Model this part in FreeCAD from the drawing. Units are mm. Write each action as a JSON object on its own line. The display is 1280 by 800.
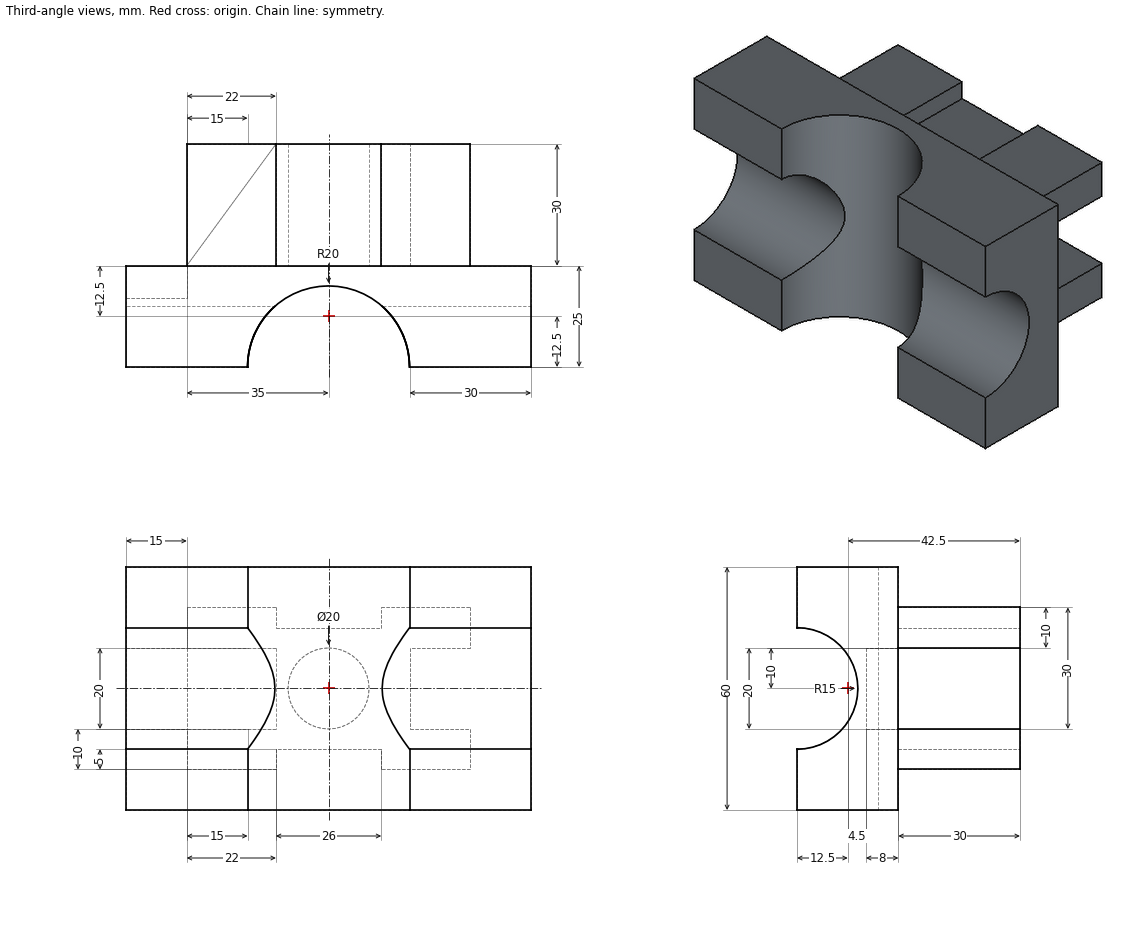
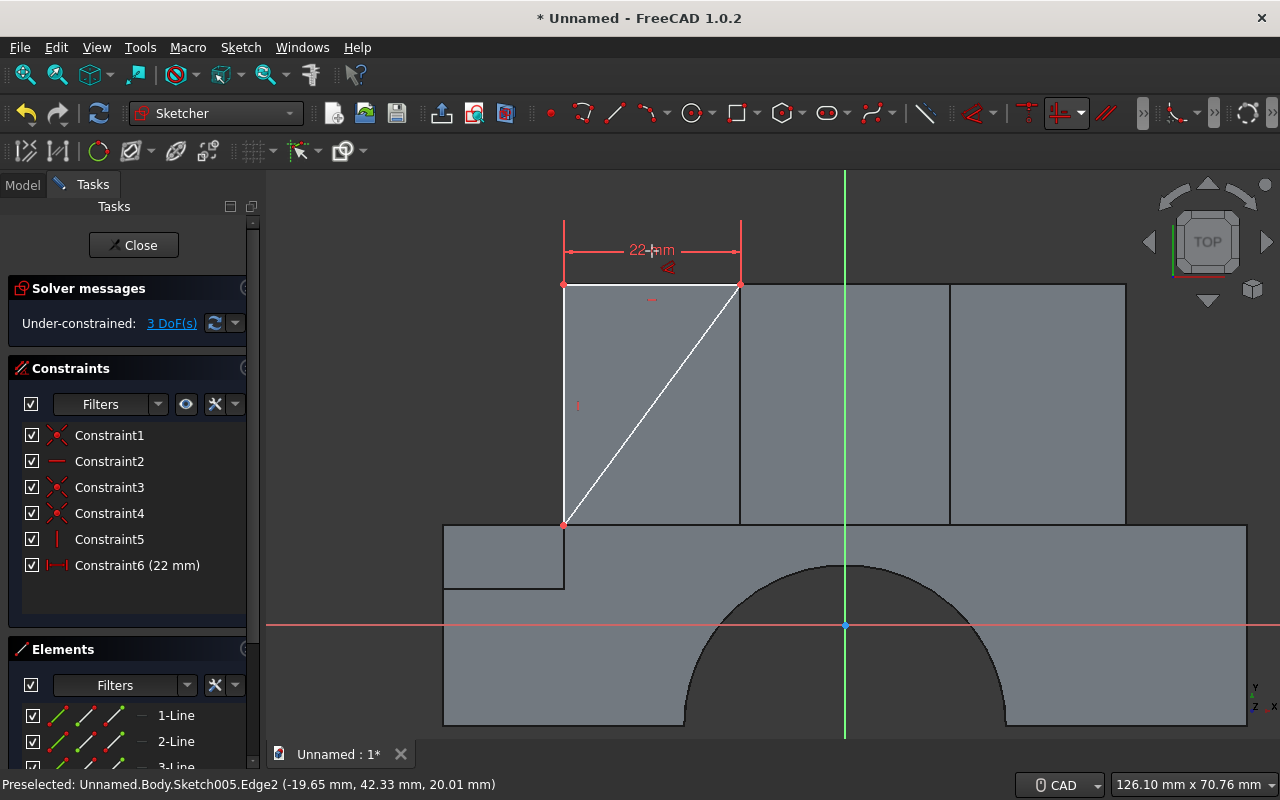
{"action": "left_click", "coordinate": [564, 357]}
{"action": "left_click", "coordinate": [530, 405]}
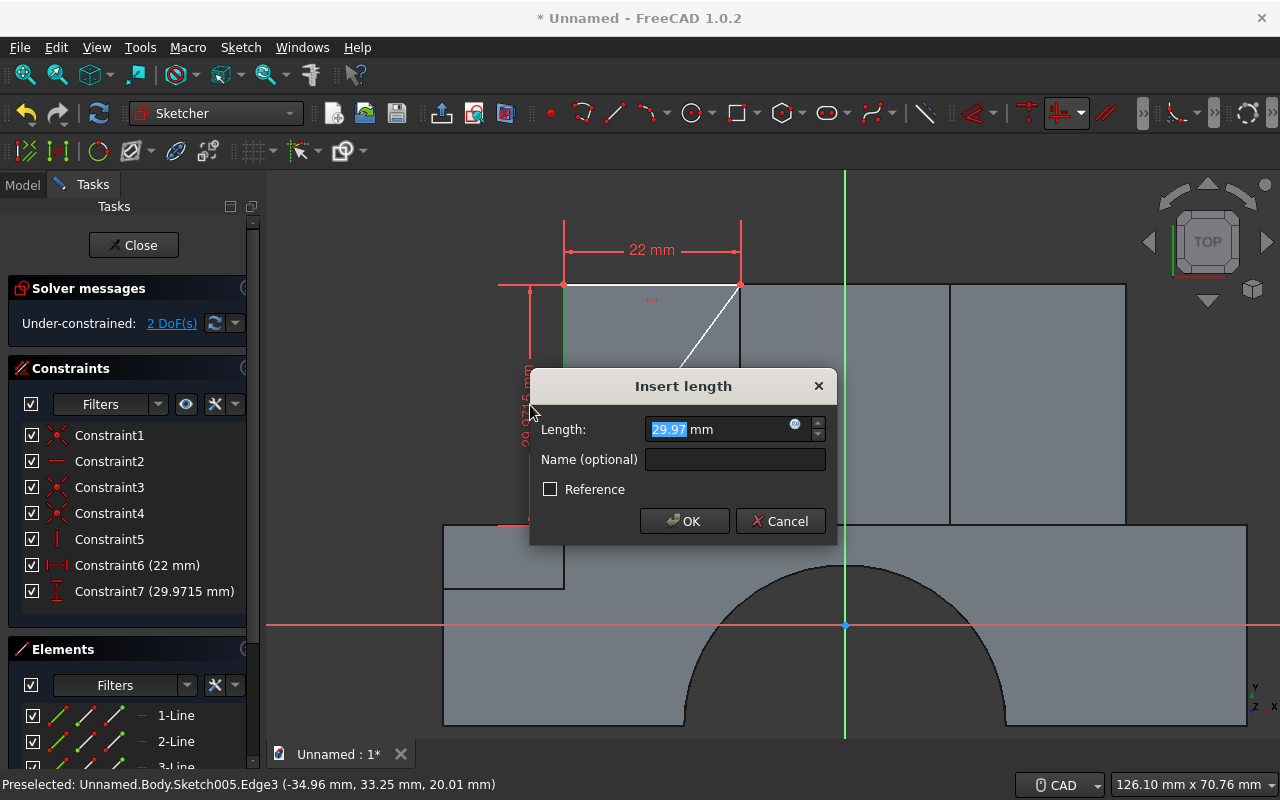
{"action": "type", "text": "30"}
{"action": "key", "text": "Return"}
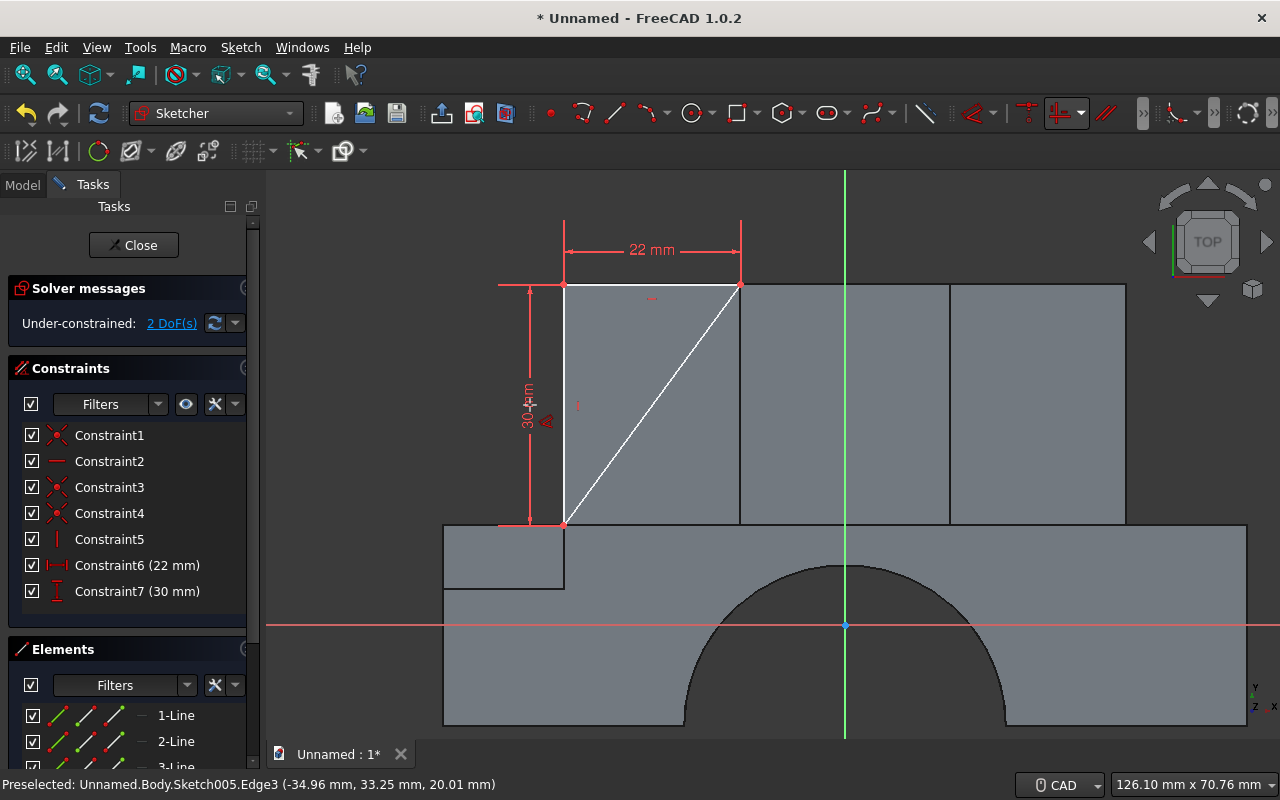
{"action": "left_click", "coordinate": [564, 526]}
{"action": "left_click", "coordinate": [704, 659]}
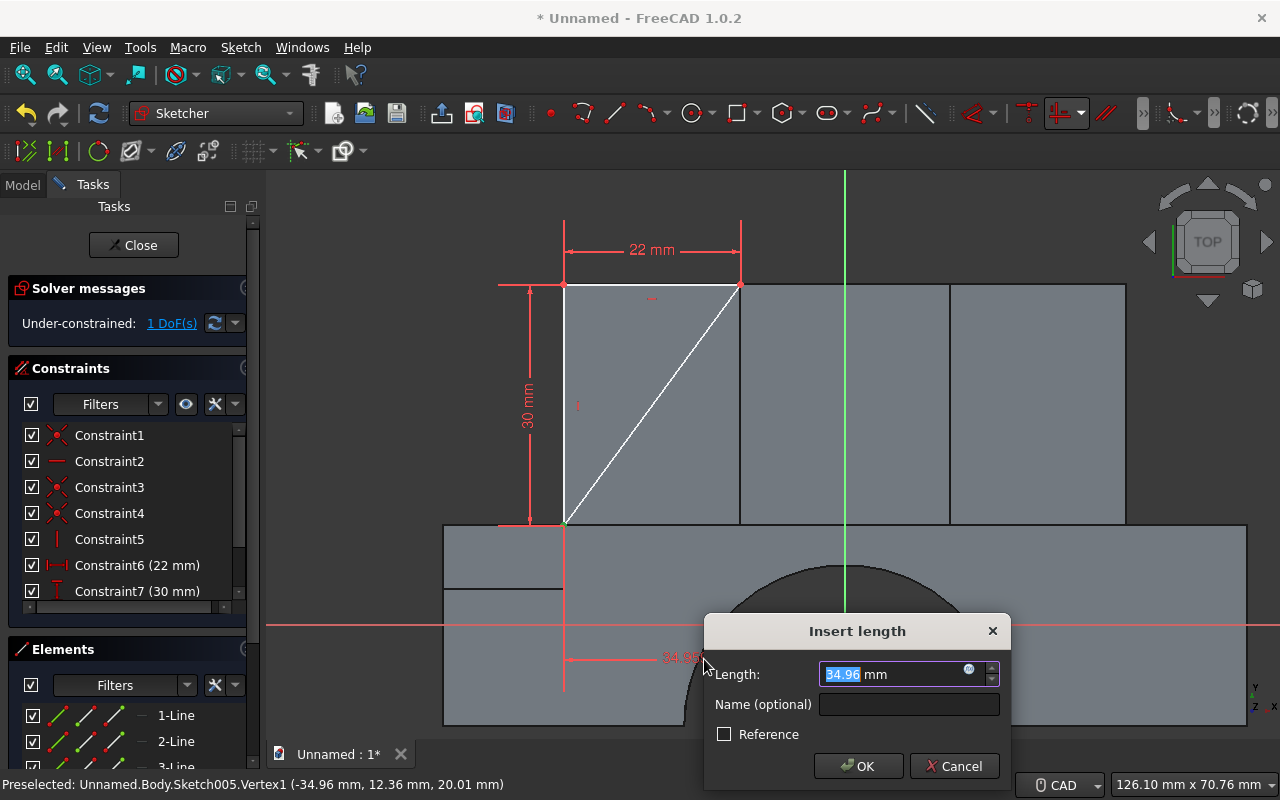
{"action": "type", "text": "35"}
{"action": "key", "text": "Return"}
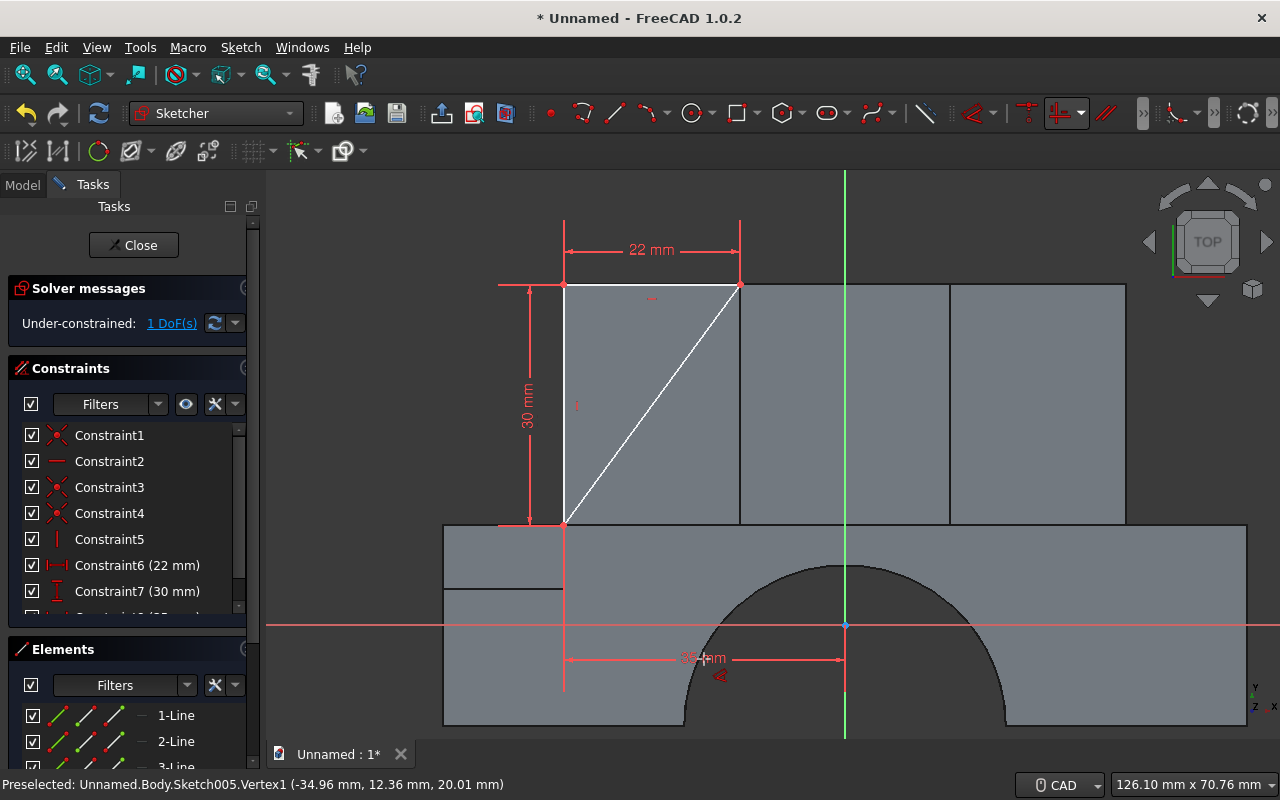
{"action": "left_click", "coordinate": [564, 526]}
{"action": "left_click", "coordinate": [879, 576]}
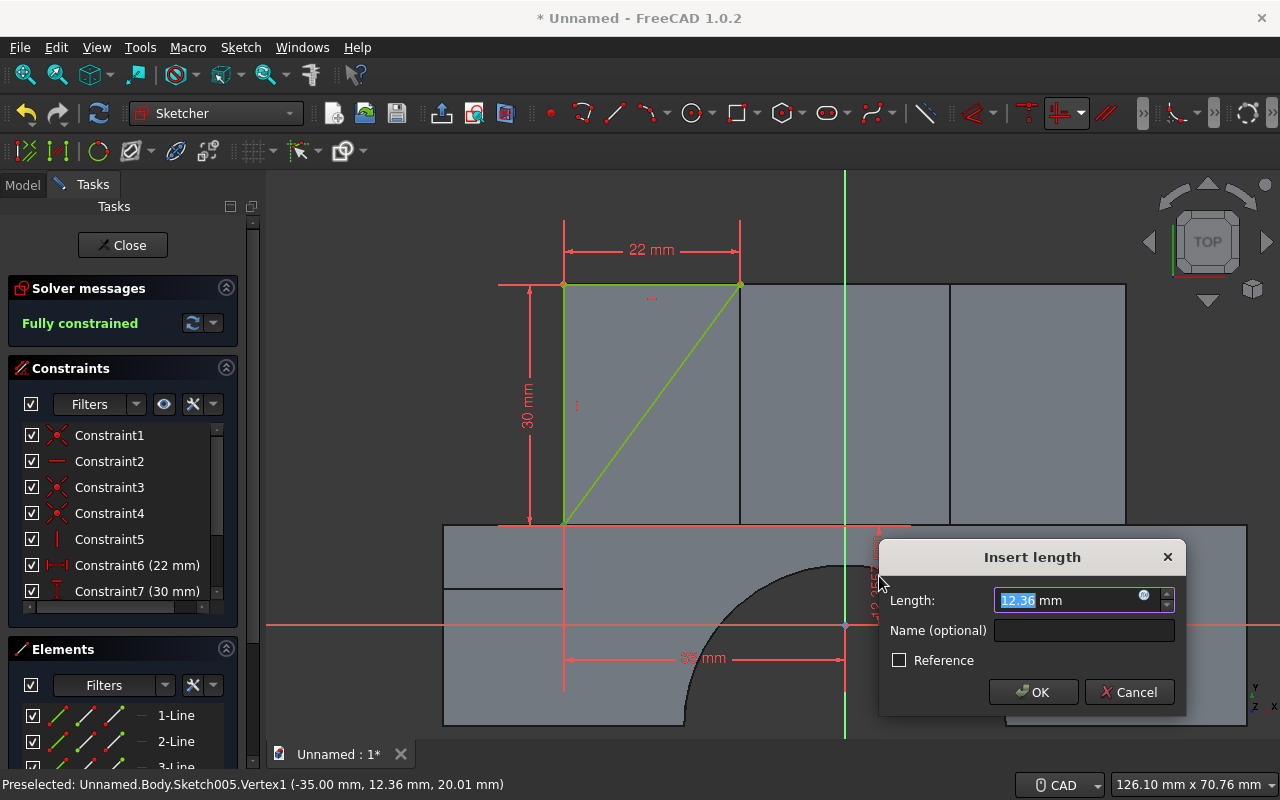
{"action": "type", "text": "12.5"}
{"action": "key", "text": "Return"}
{"action": "key", "text": "Escape"}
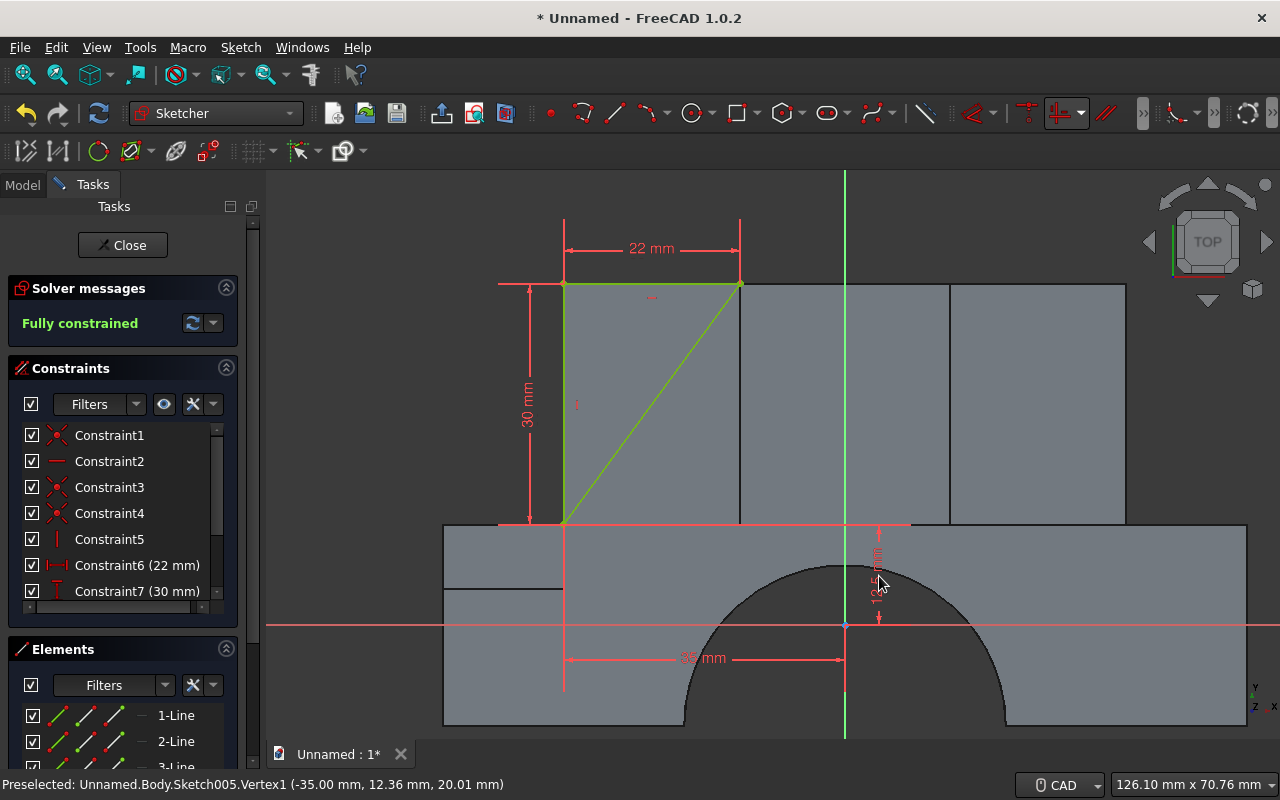
{"action": "left_click", "coordinate": [123, 245]}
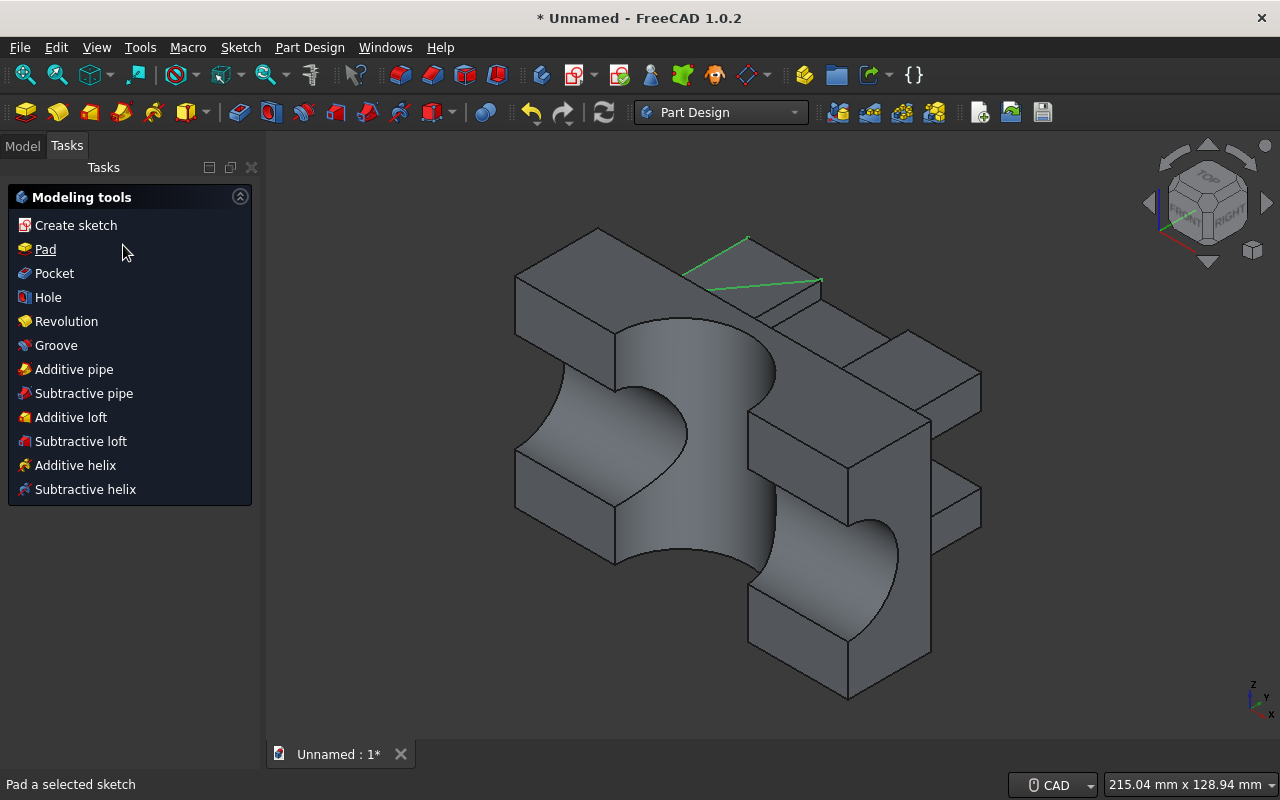
{"action": "left_click", "coordinate": [240, 112]}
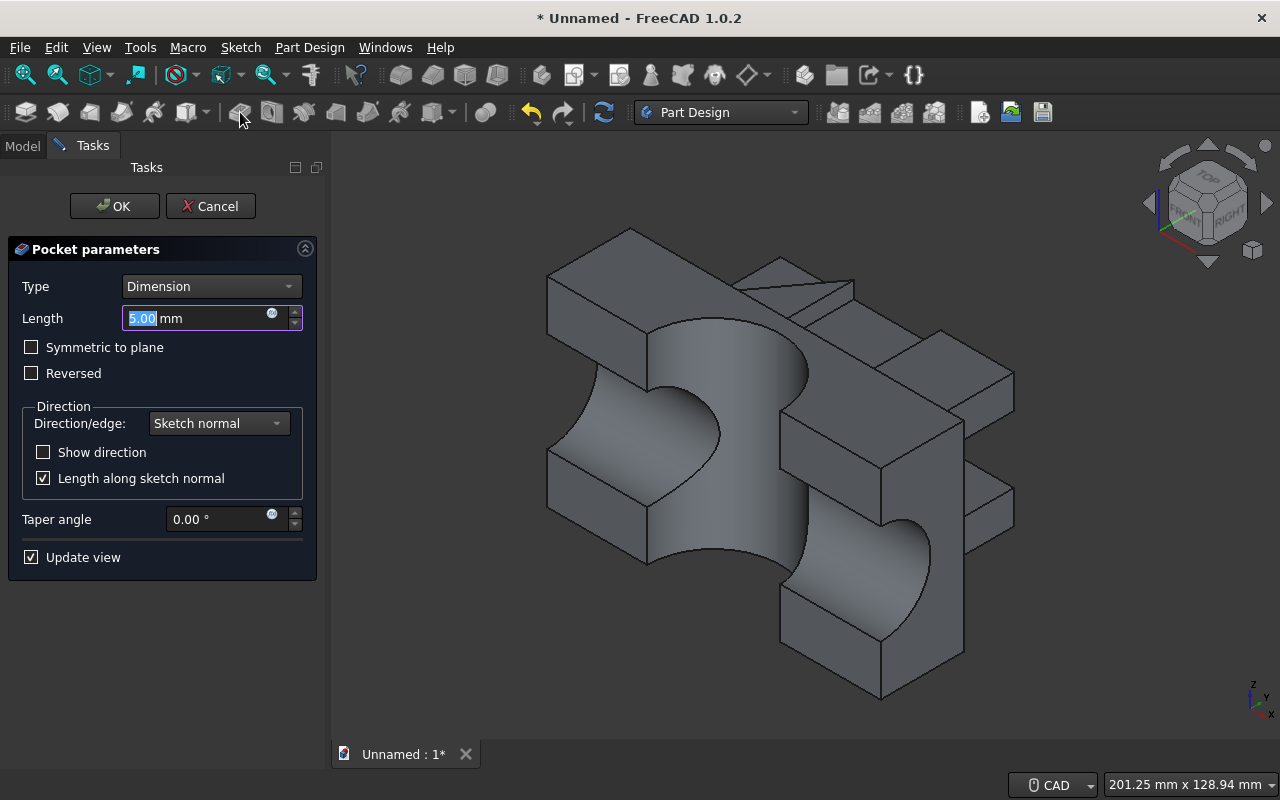
{"action": "type", "text": "30"}
{"action": "key", "text": "Tab"}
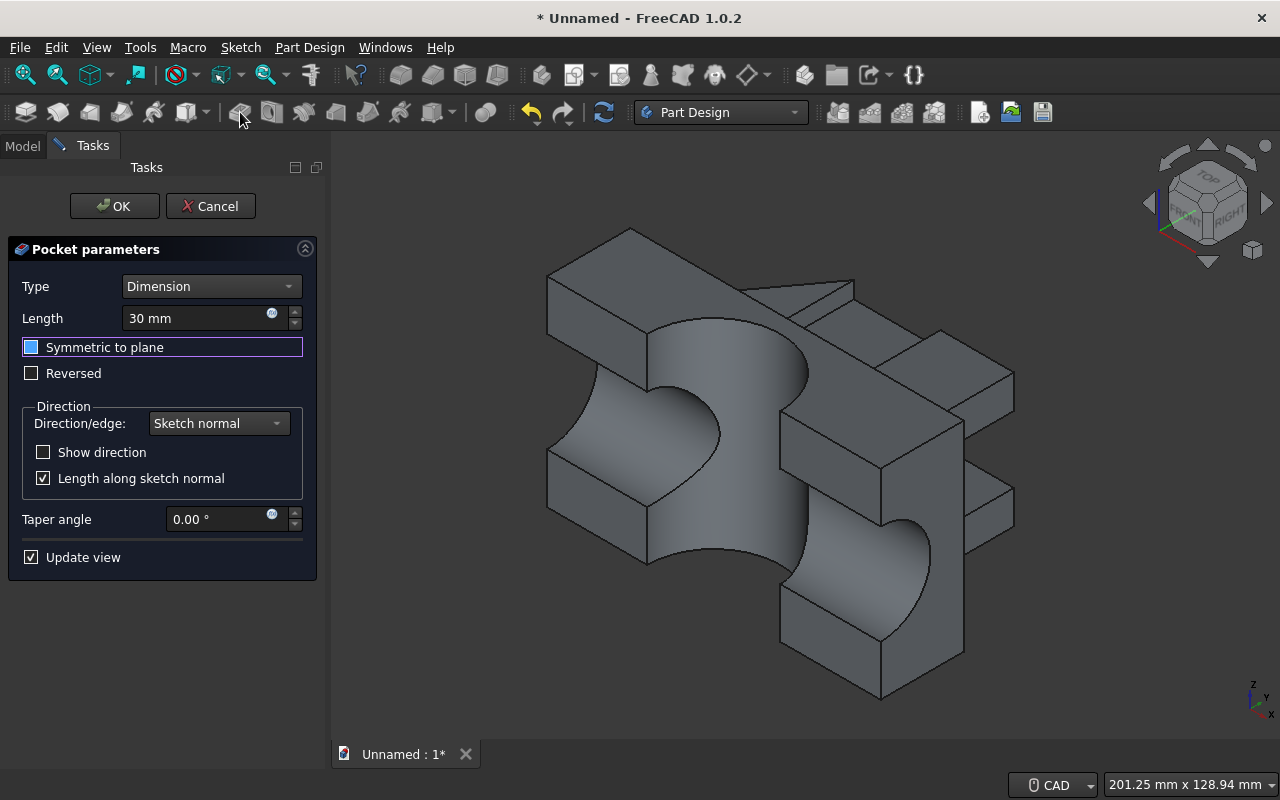
{"action": "left_click", "coordinate": [115, 206]}